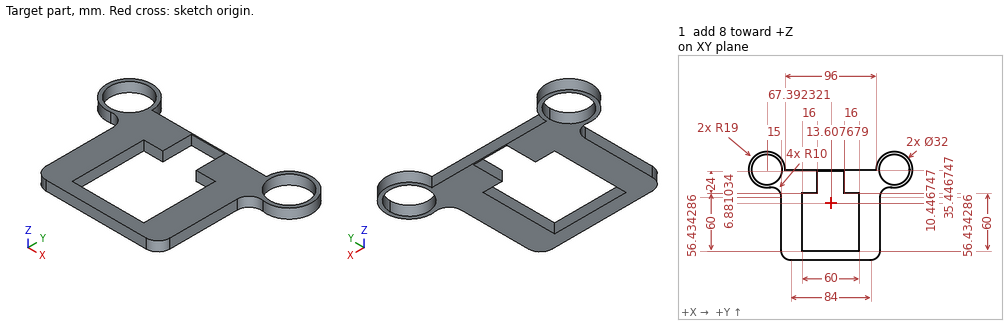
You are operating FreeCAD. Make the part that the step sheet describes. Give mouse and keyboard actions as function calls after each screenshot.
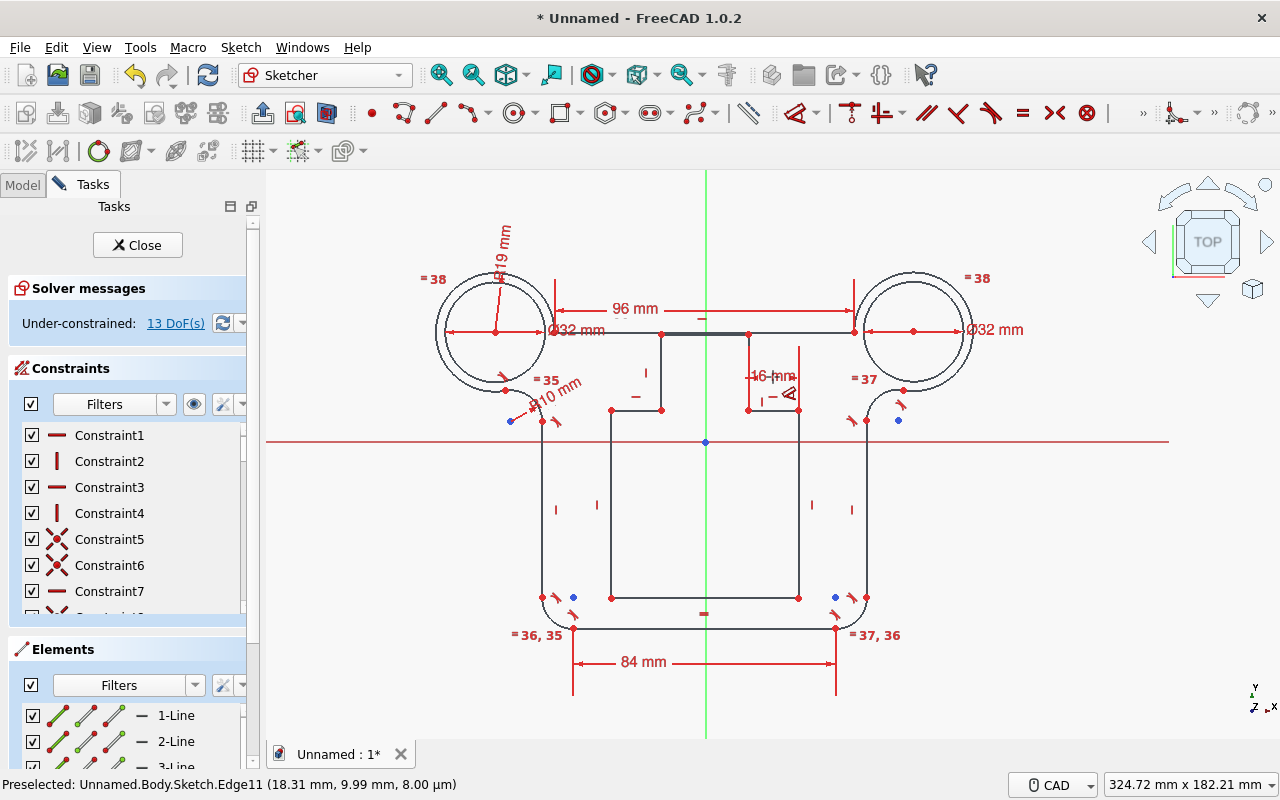
click(799, 467)
click(833, 504)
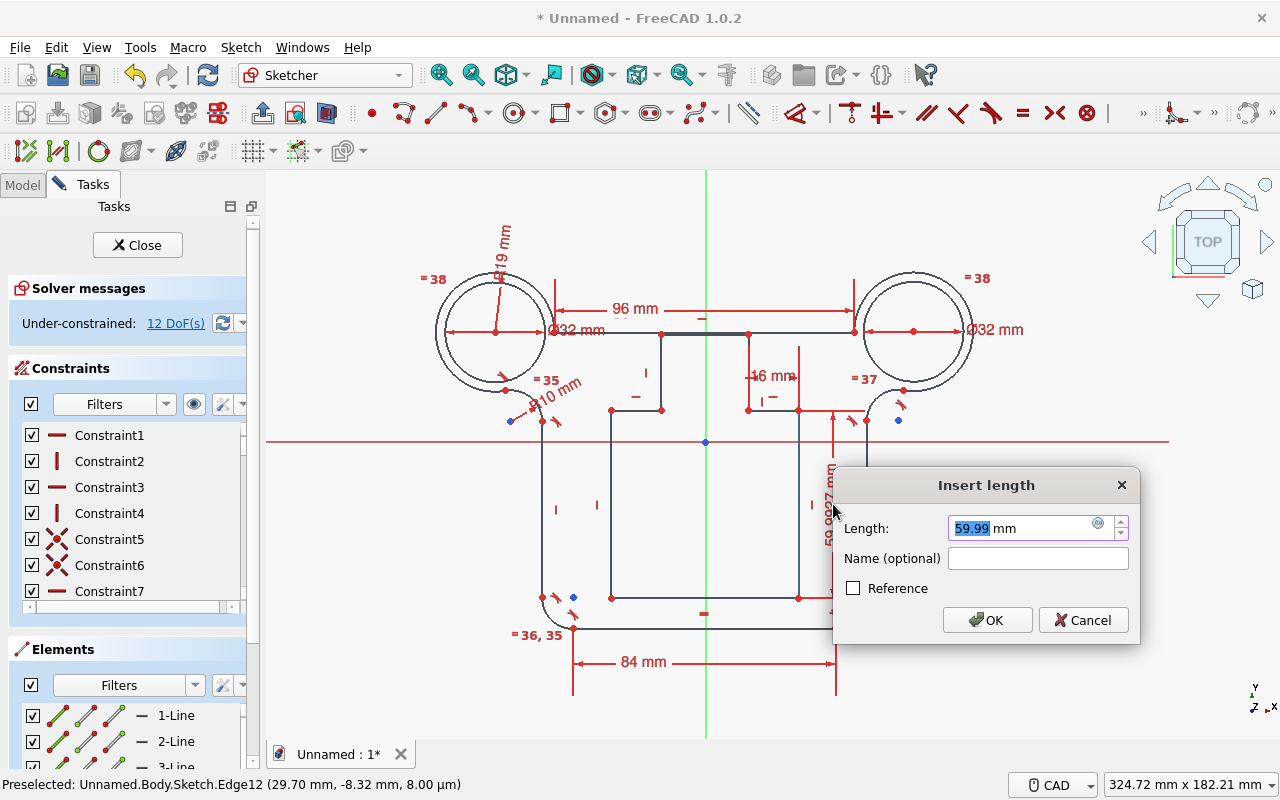
text(60)
key(Return)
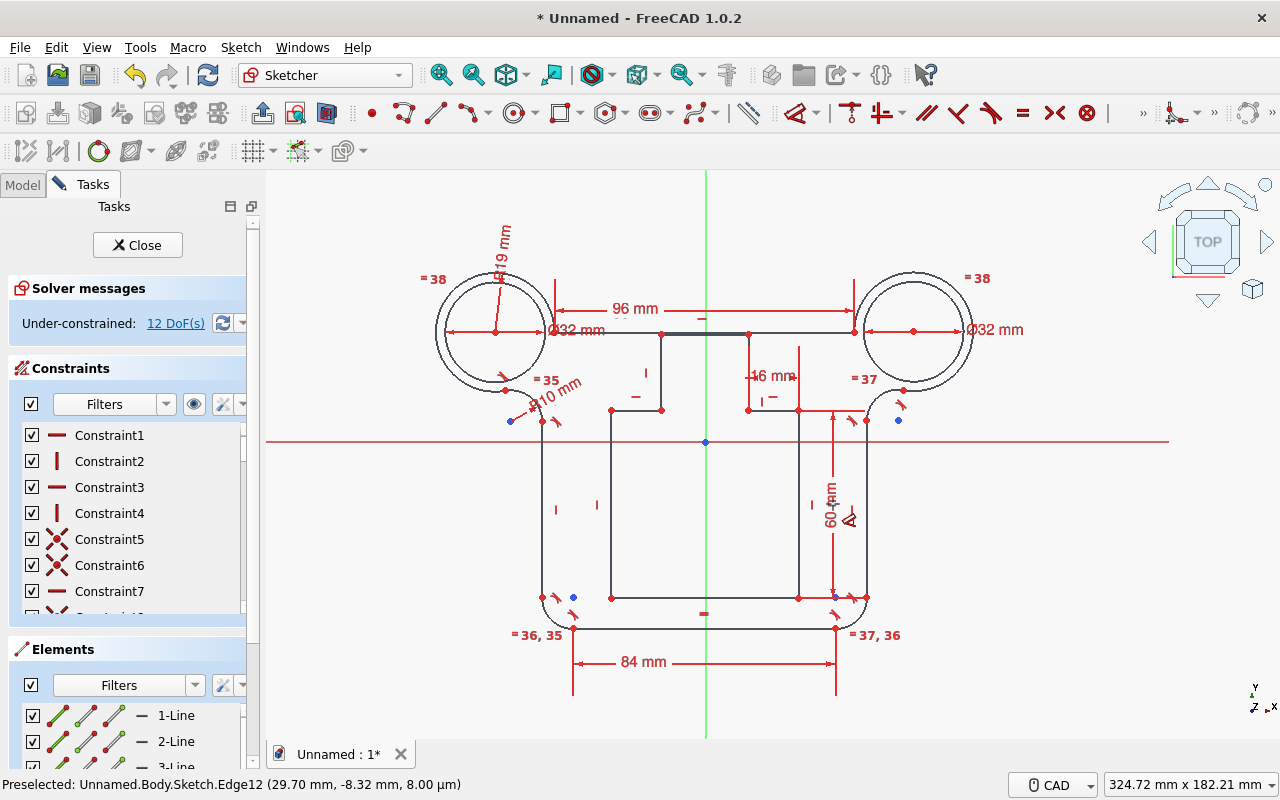
click(742, 598)
click(662, 564)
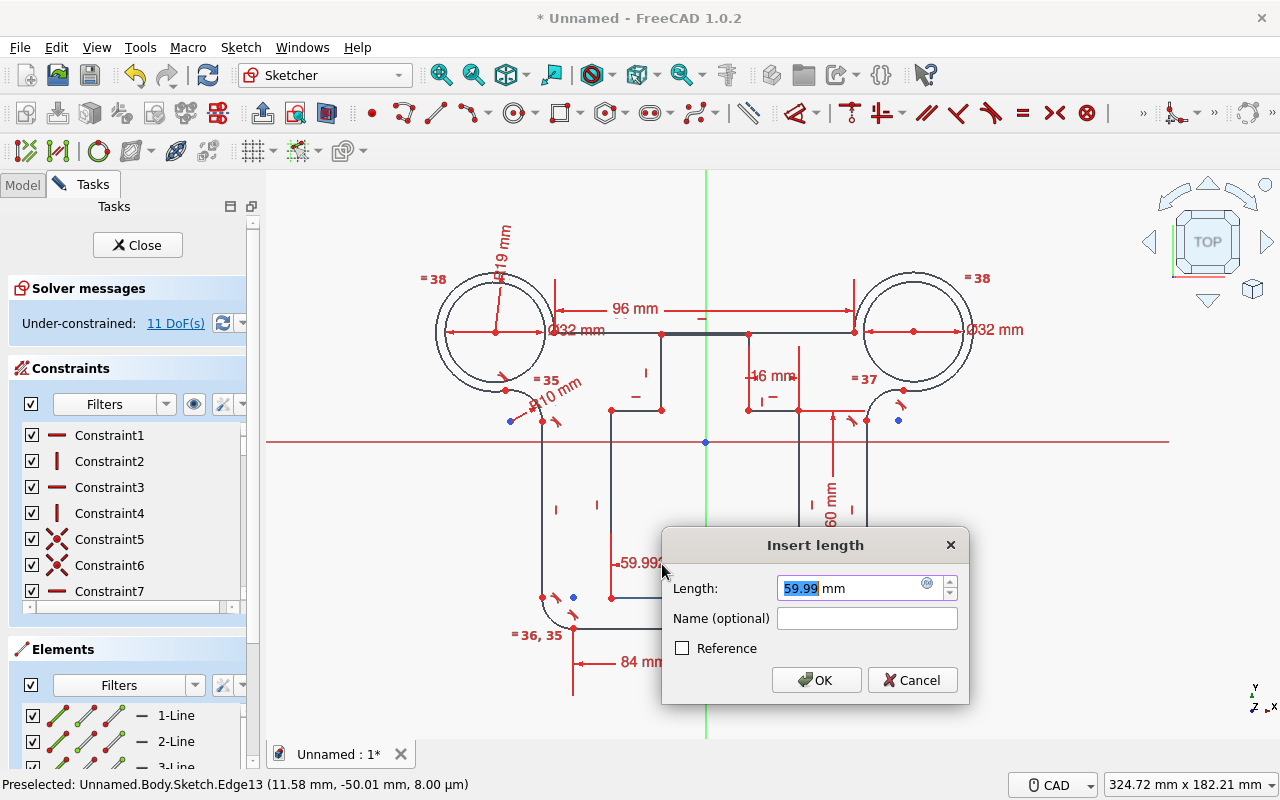
text(60)
key(Return)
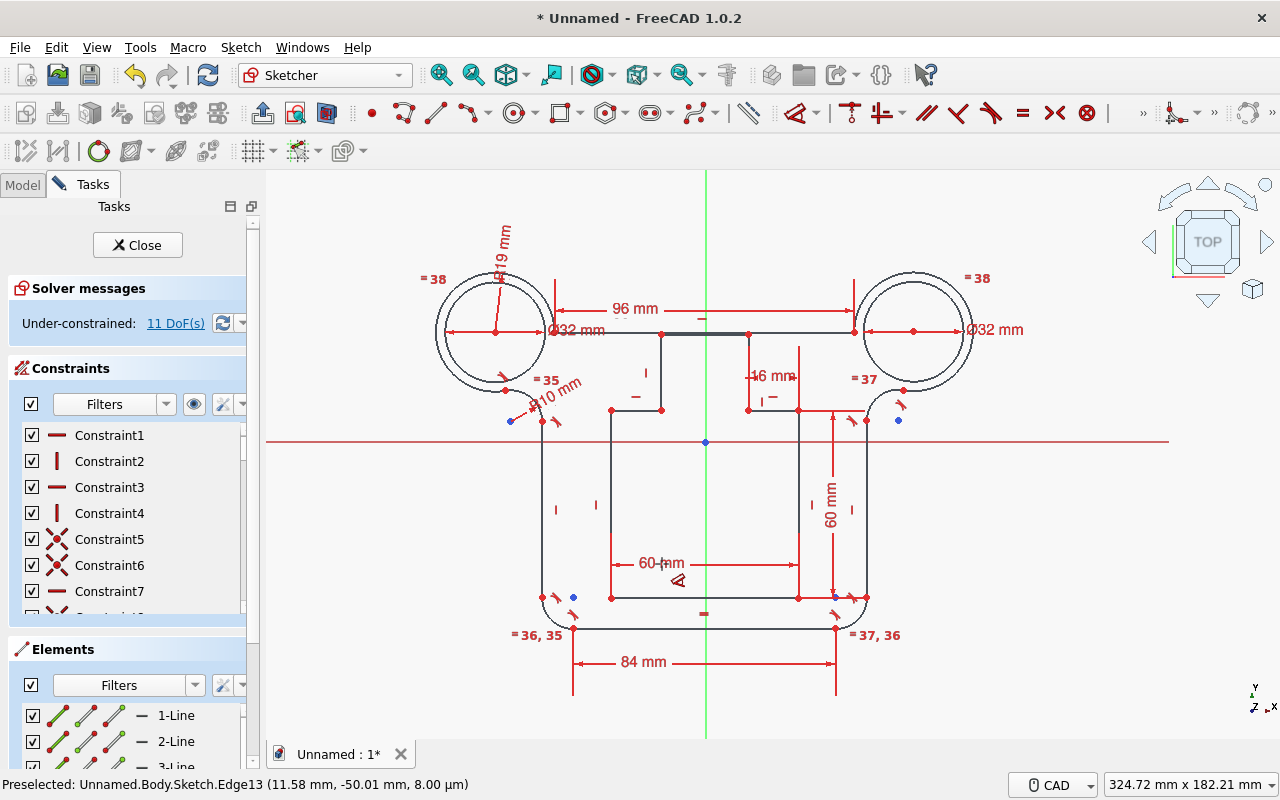
click(611, 542)
click(577, 504)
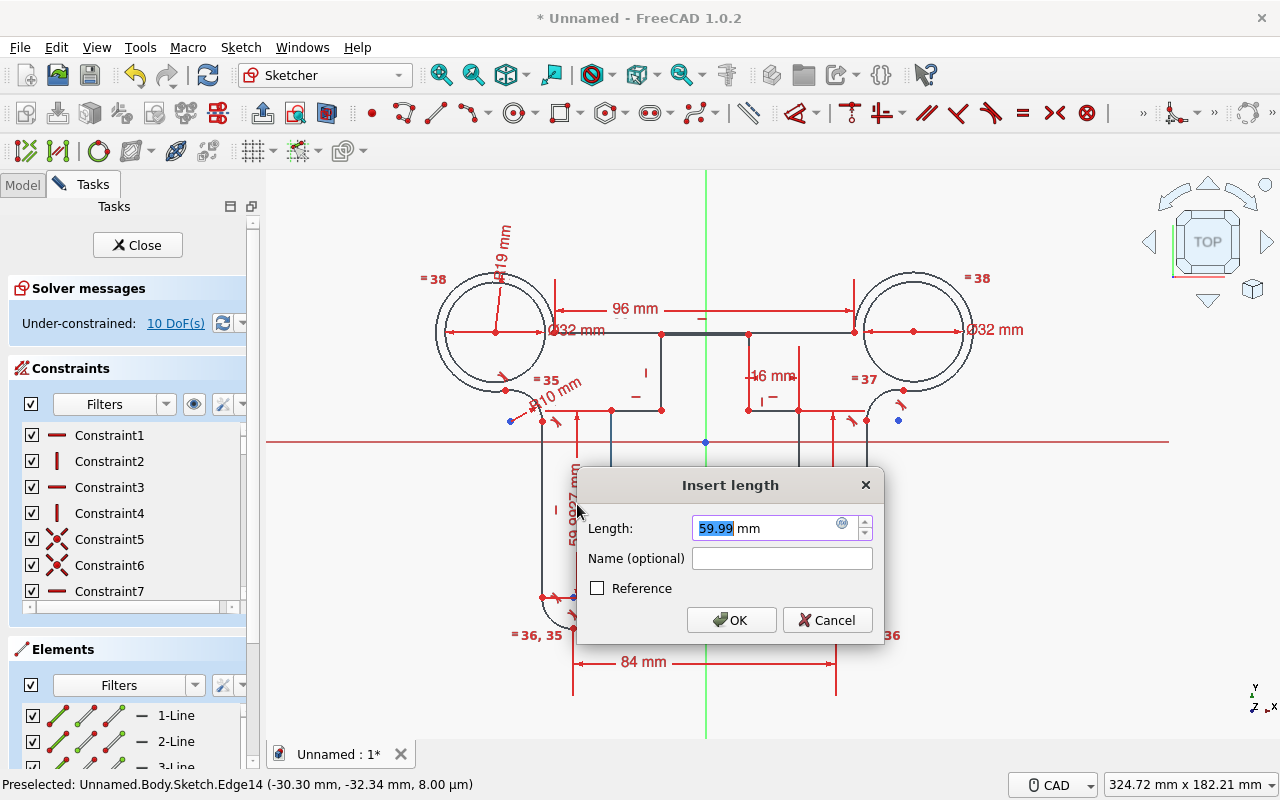
text(60)
key(Return)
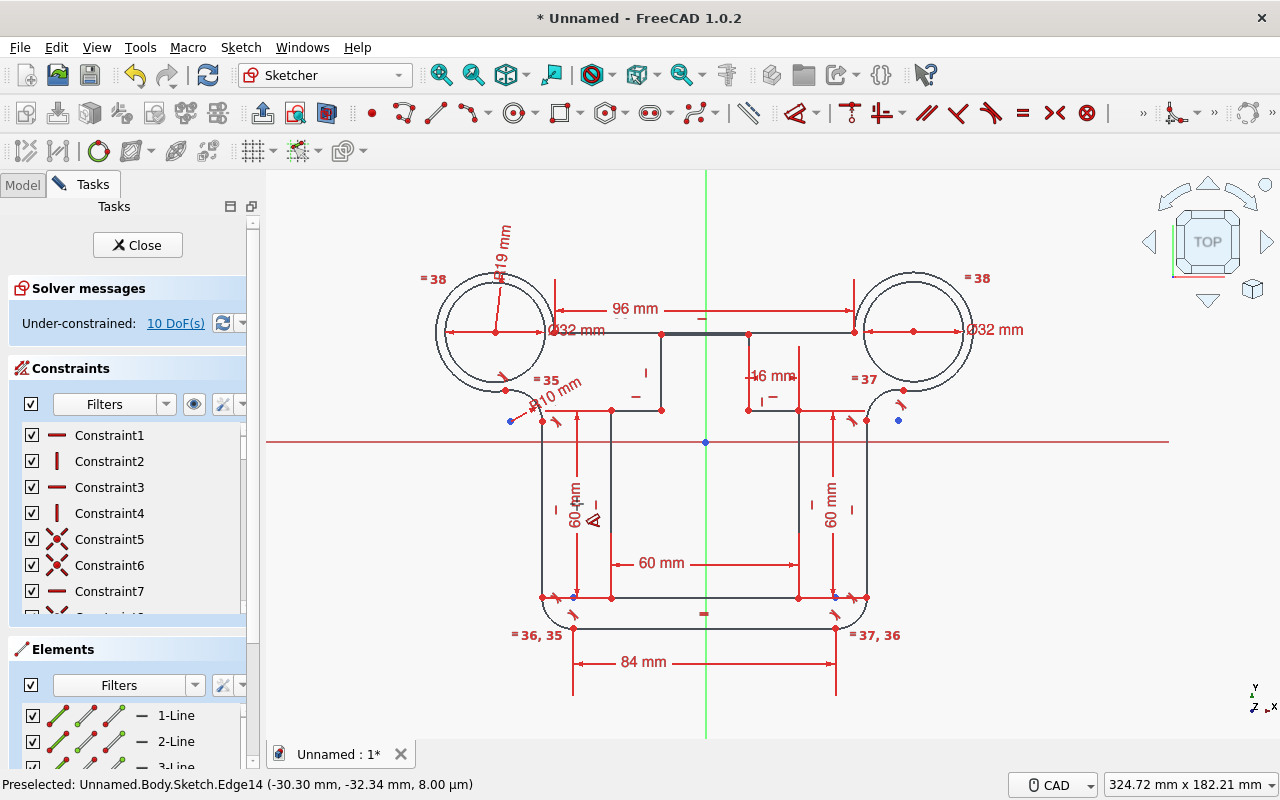
click(626, 411)
click(636, 377)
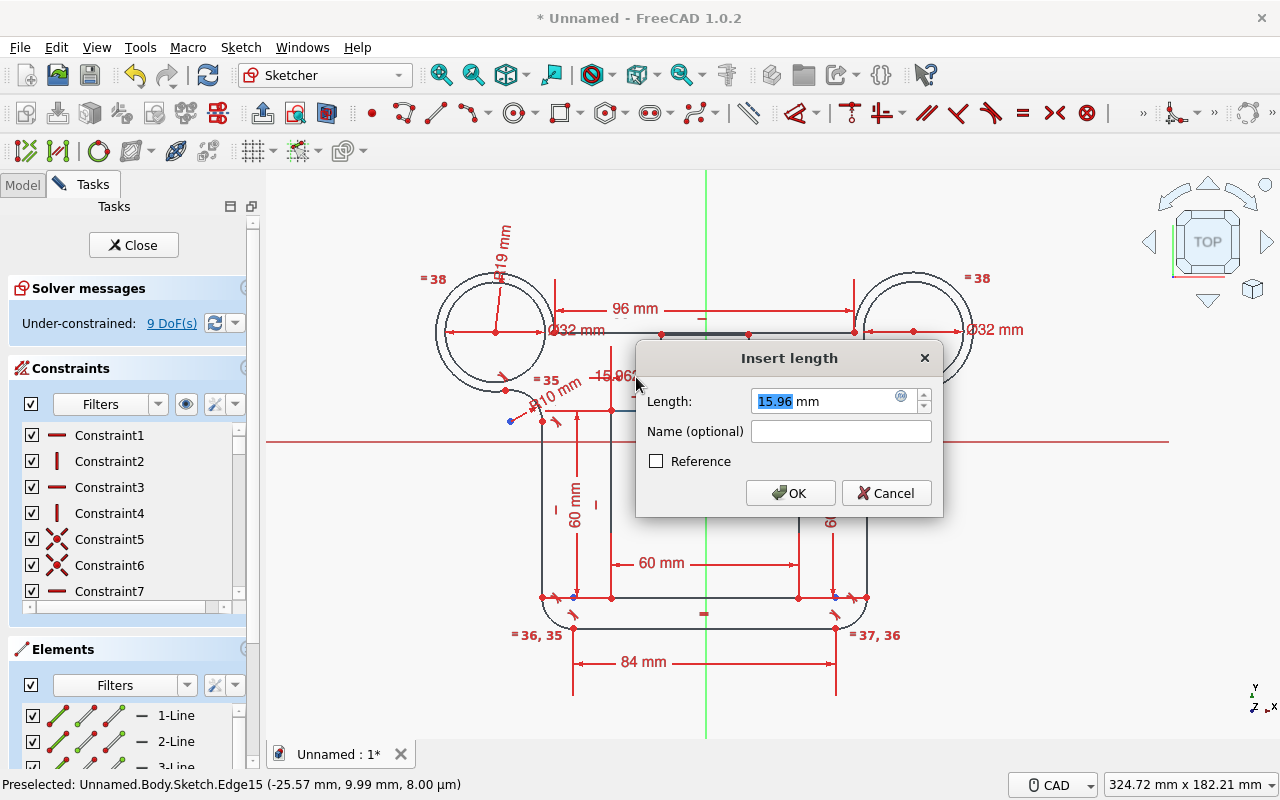
text(16)
key(Return)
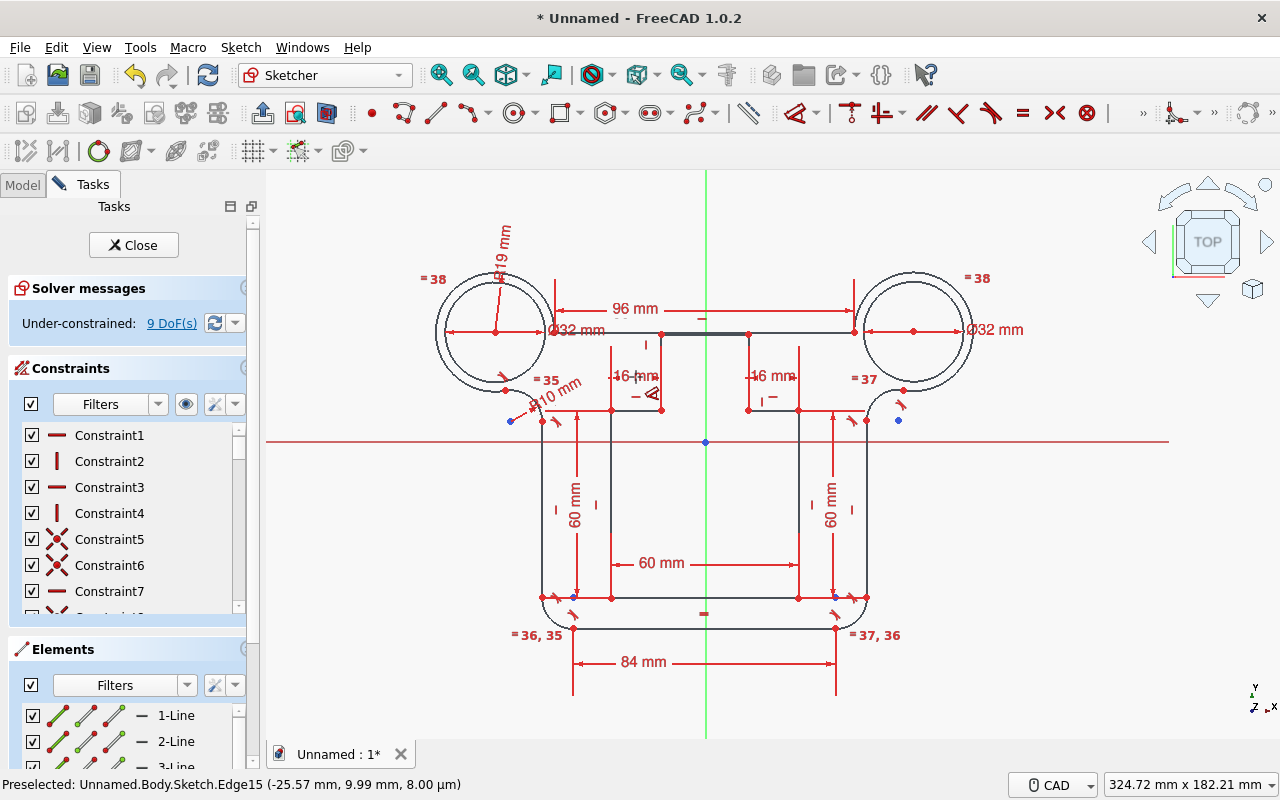
click(661, 388)
click(627, 355)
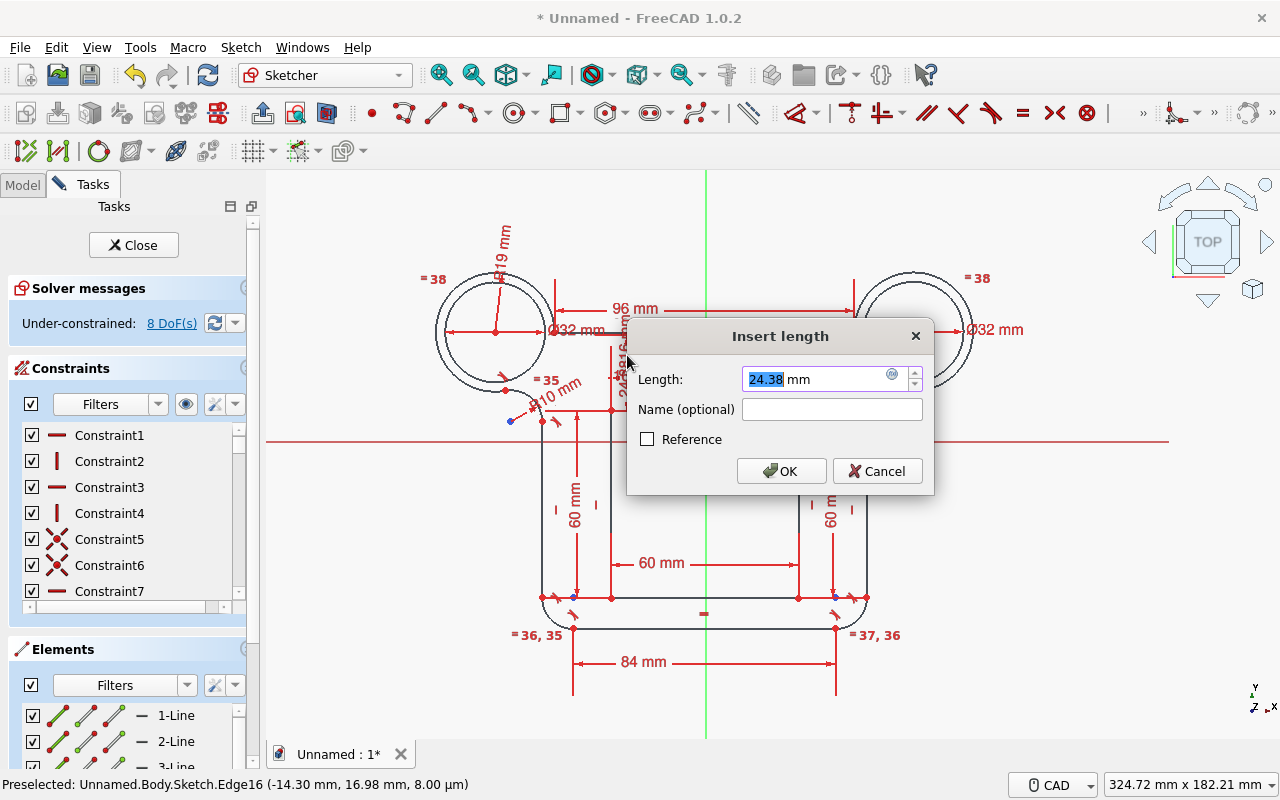
text(24)
key(Return)